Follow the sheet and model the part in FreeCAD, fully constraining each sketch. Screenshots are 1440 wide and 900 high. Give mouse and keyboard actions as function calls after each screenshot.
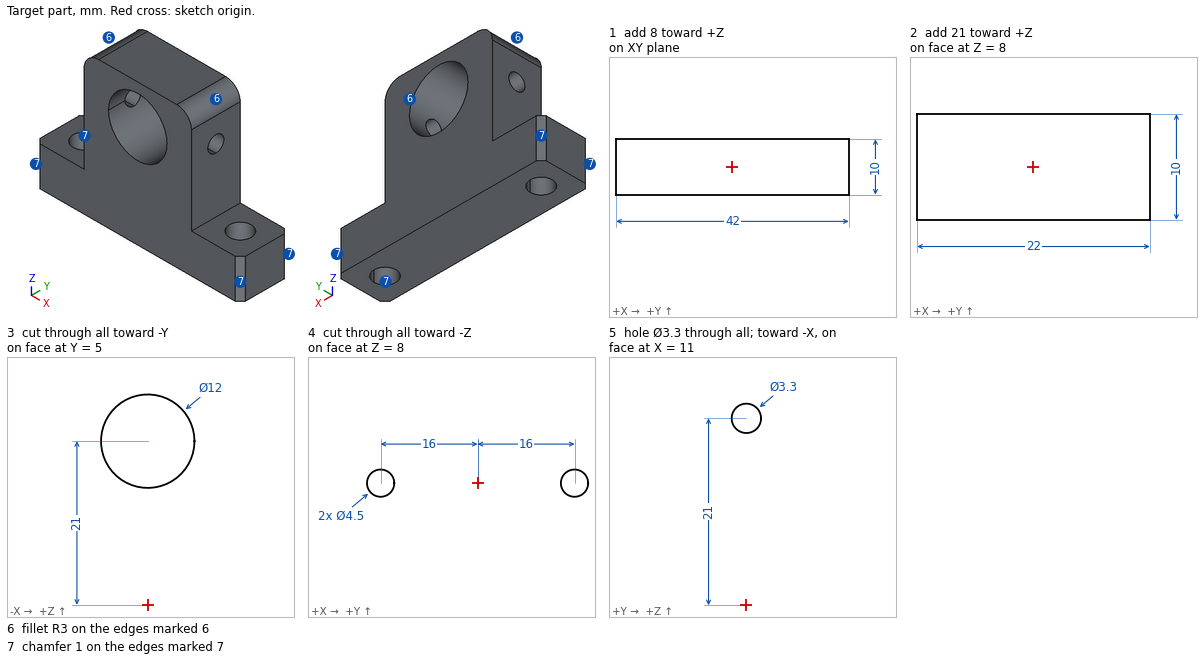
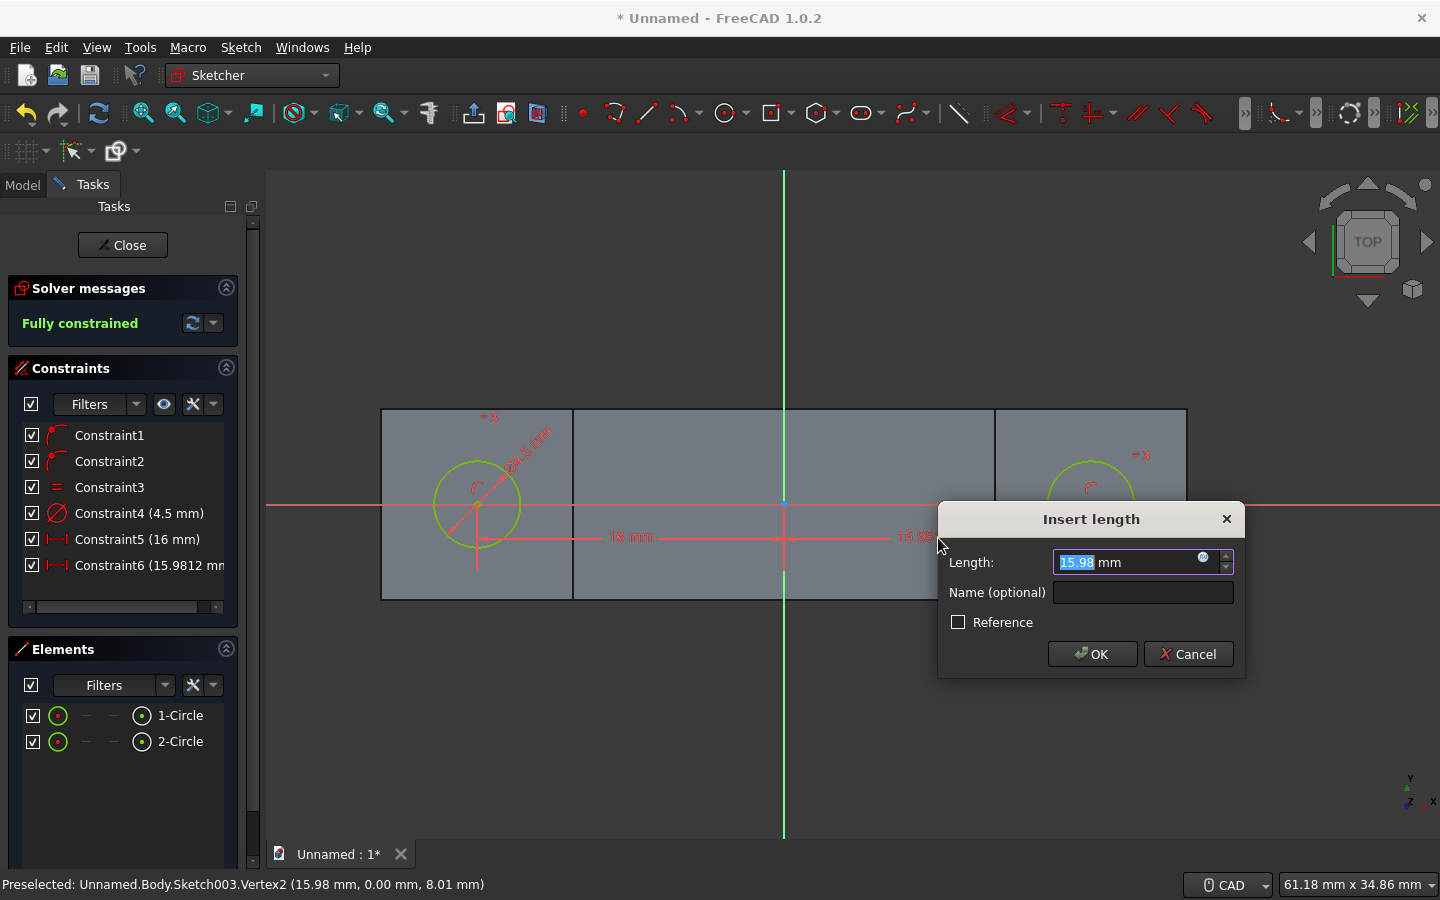
text(16)
key(Return)
key(Escape)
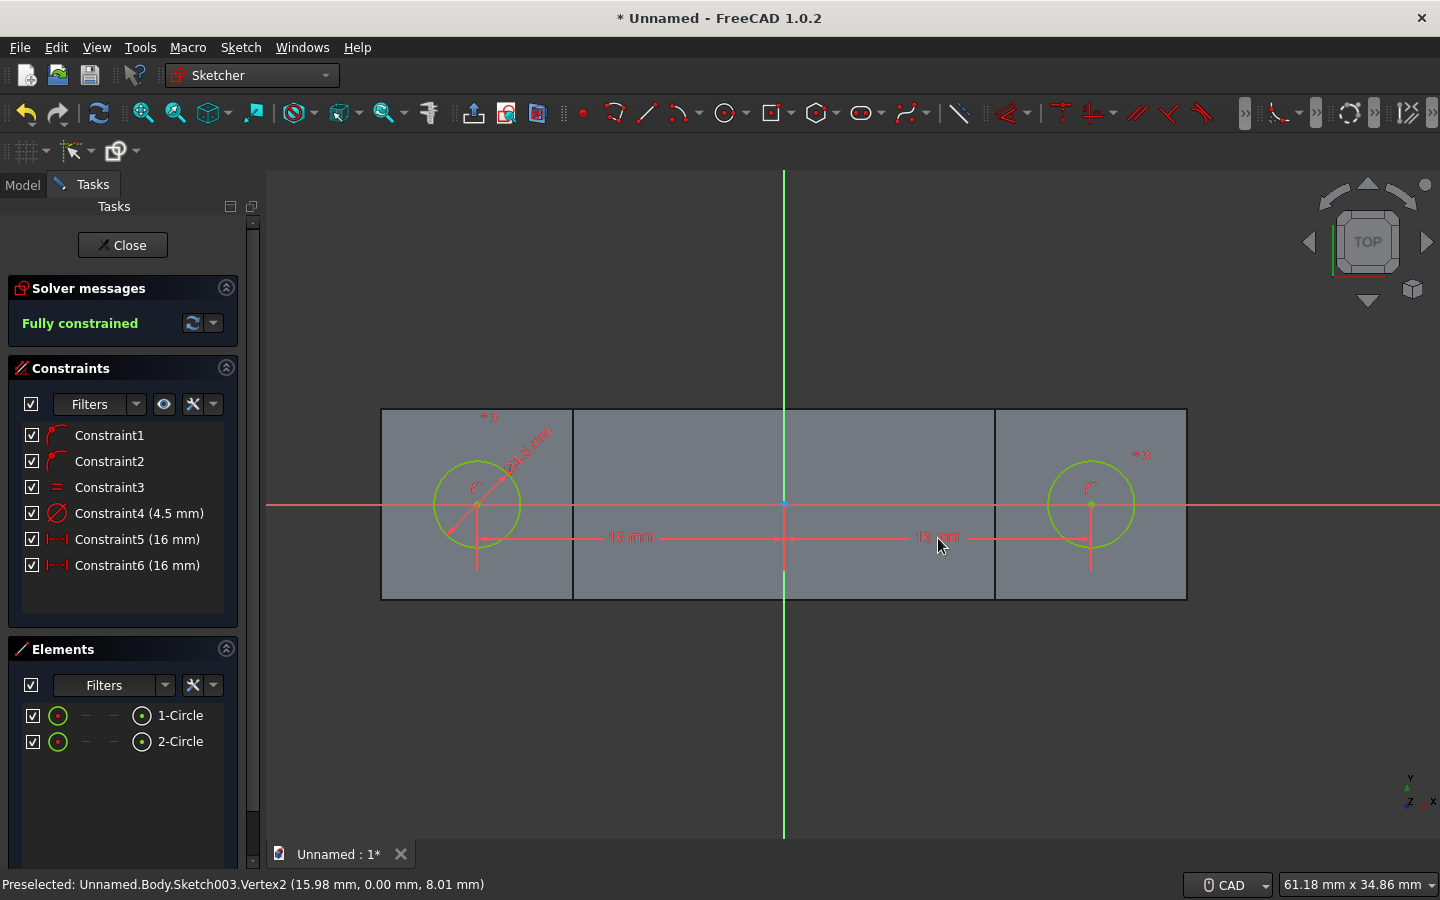
click(123, 245)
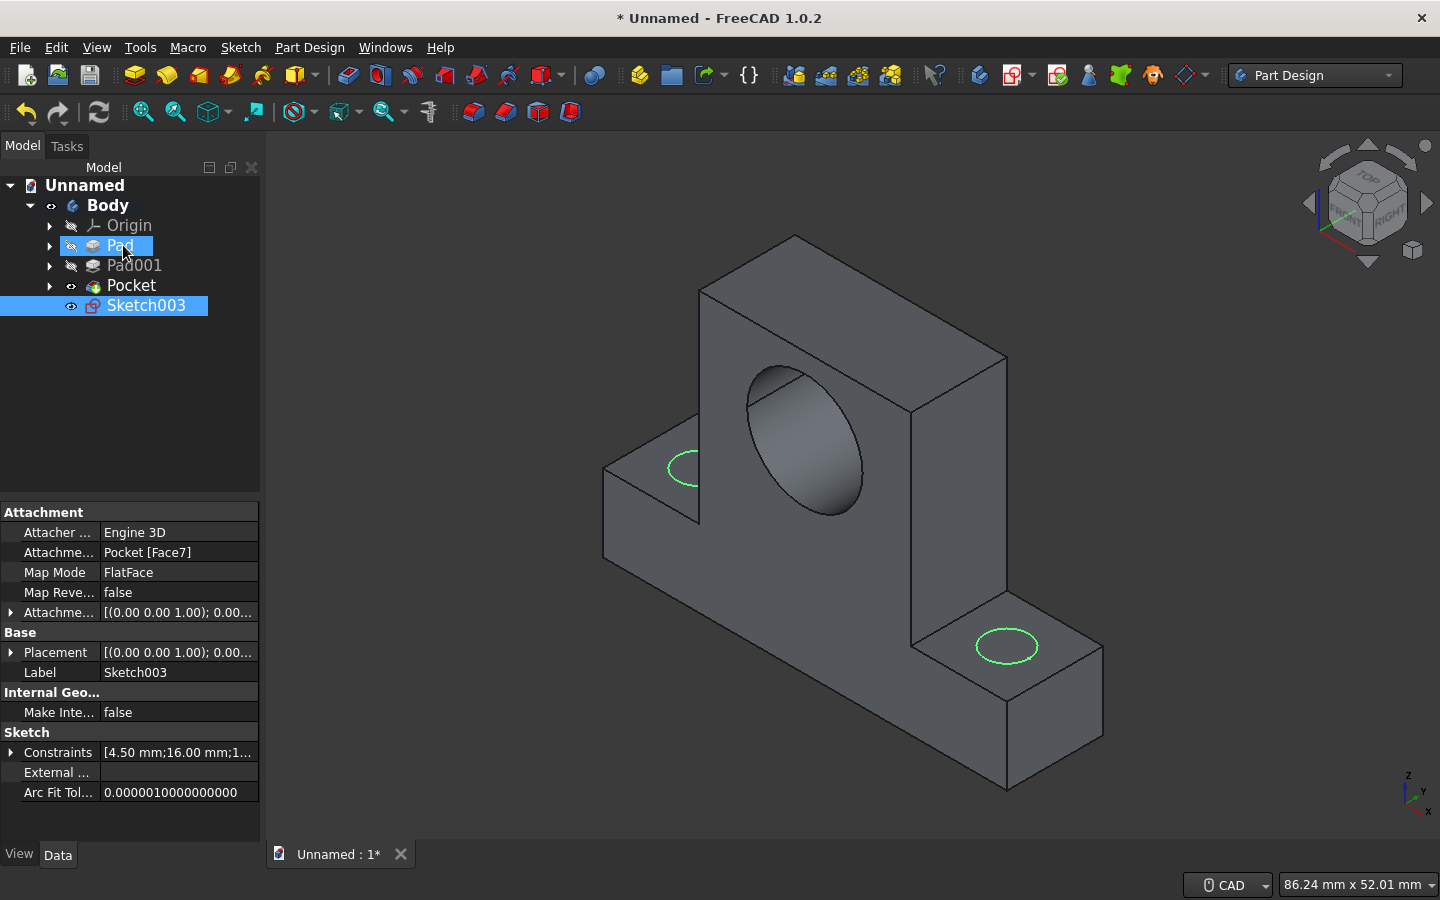
click(350, 76)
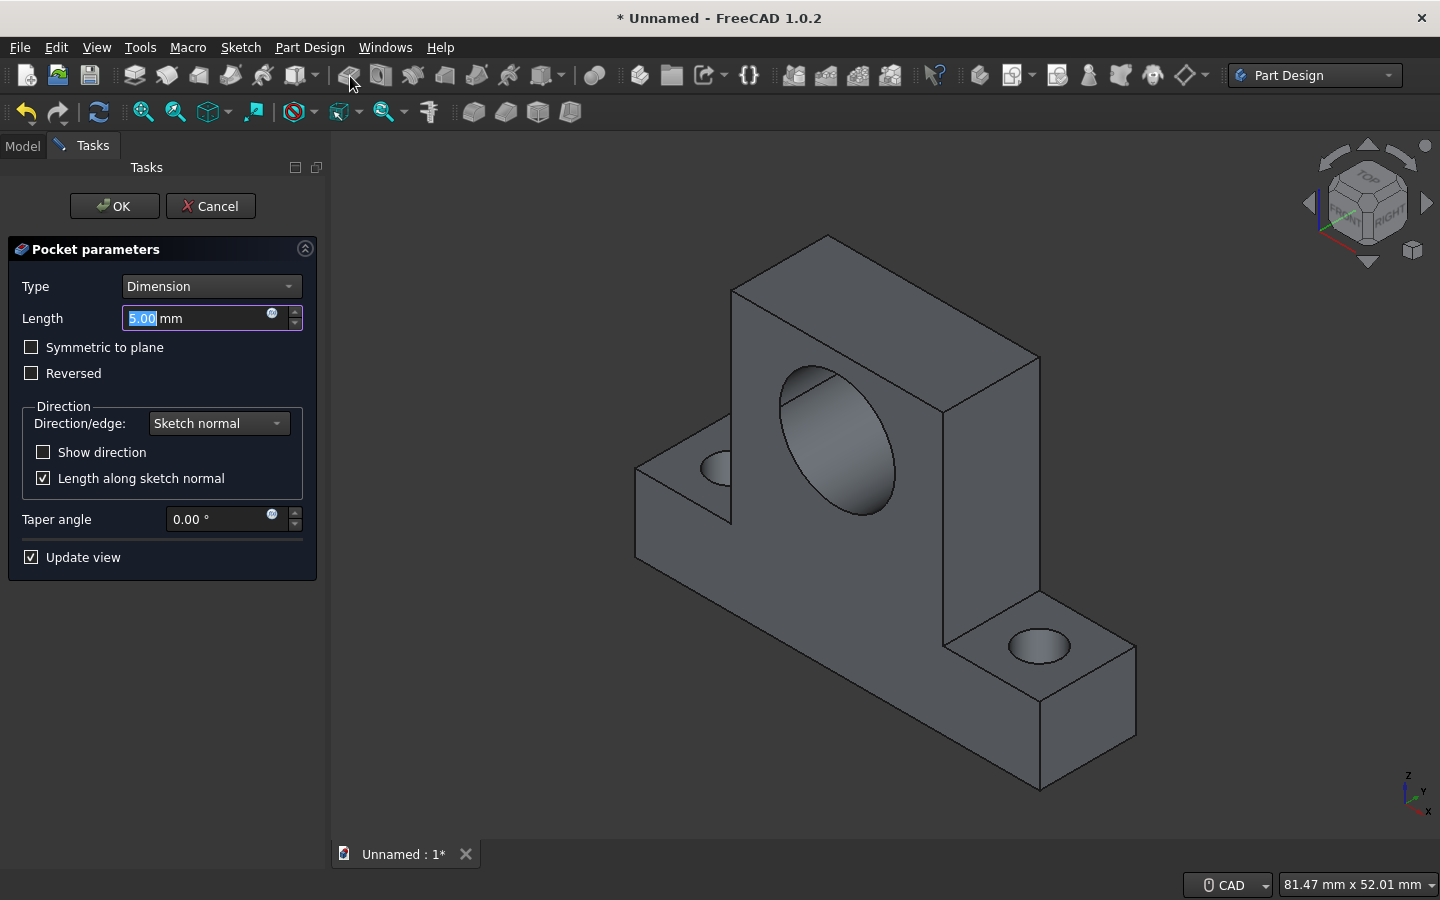
click(212, 286)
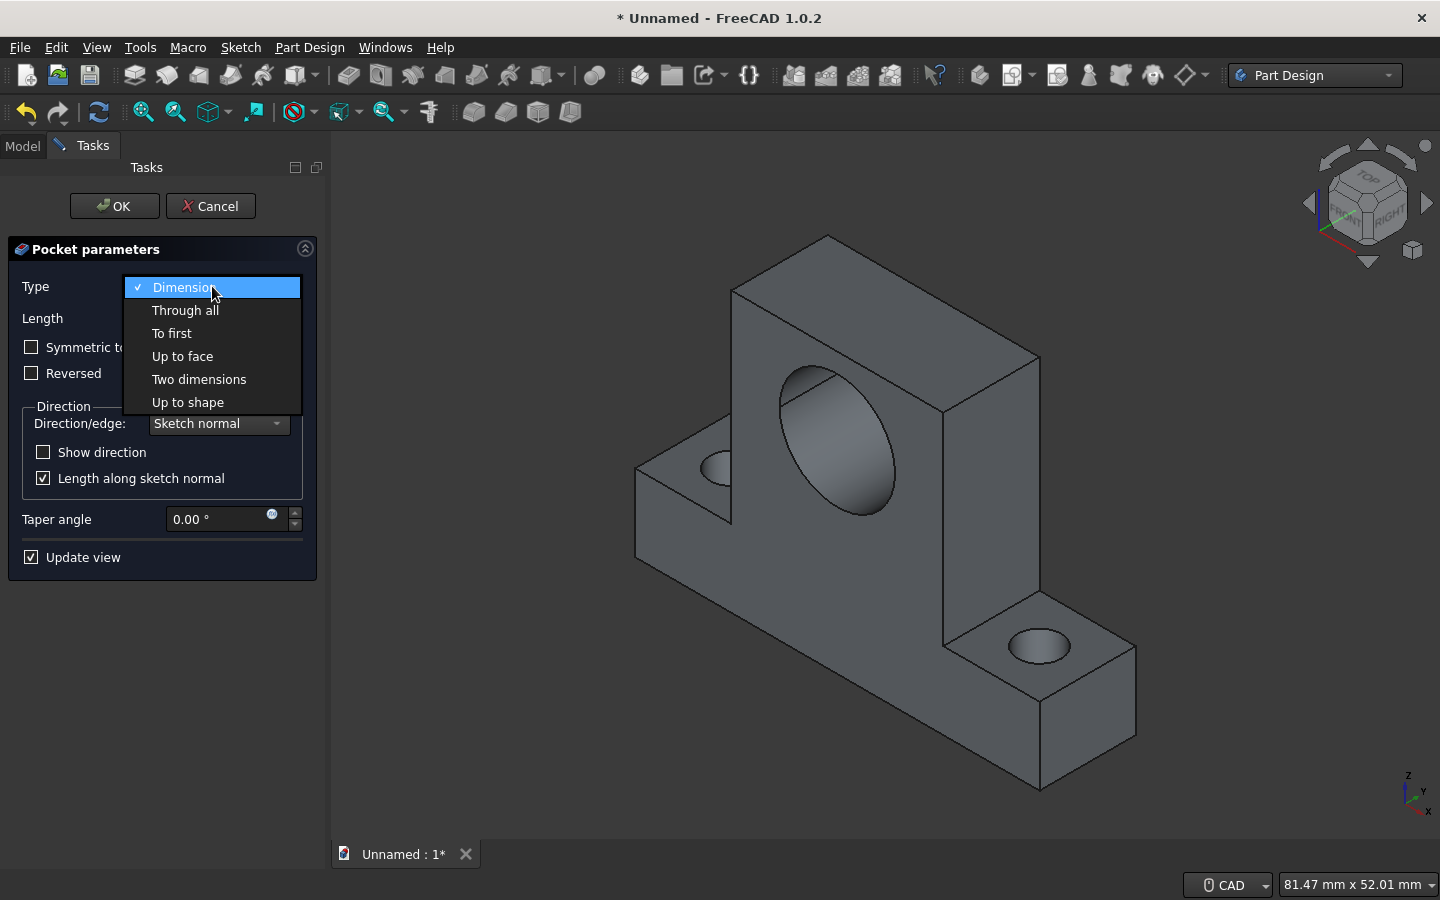
click(212, 310)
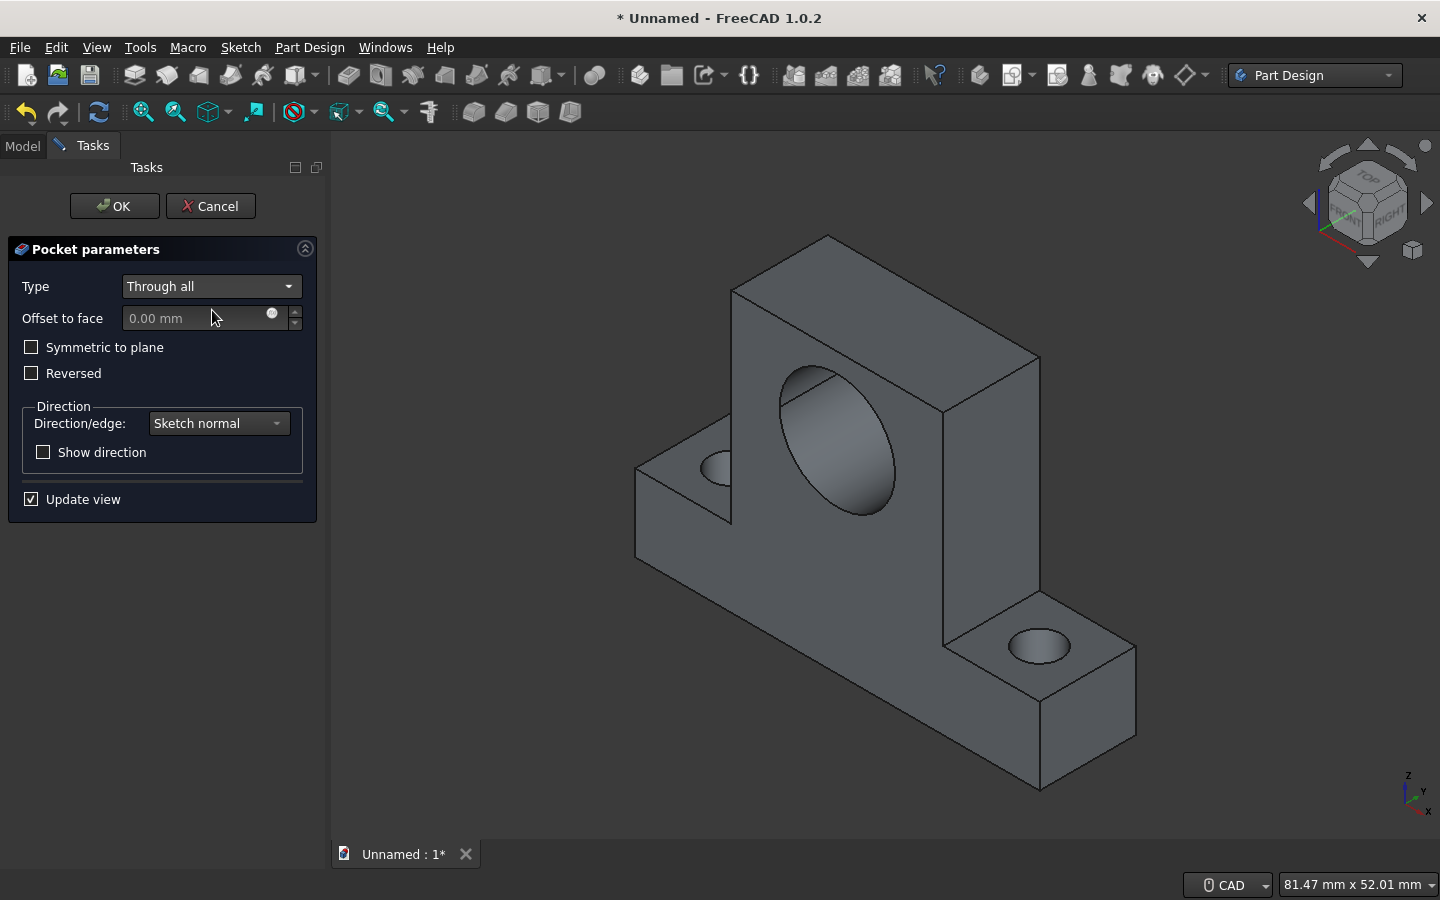
click(115, 206)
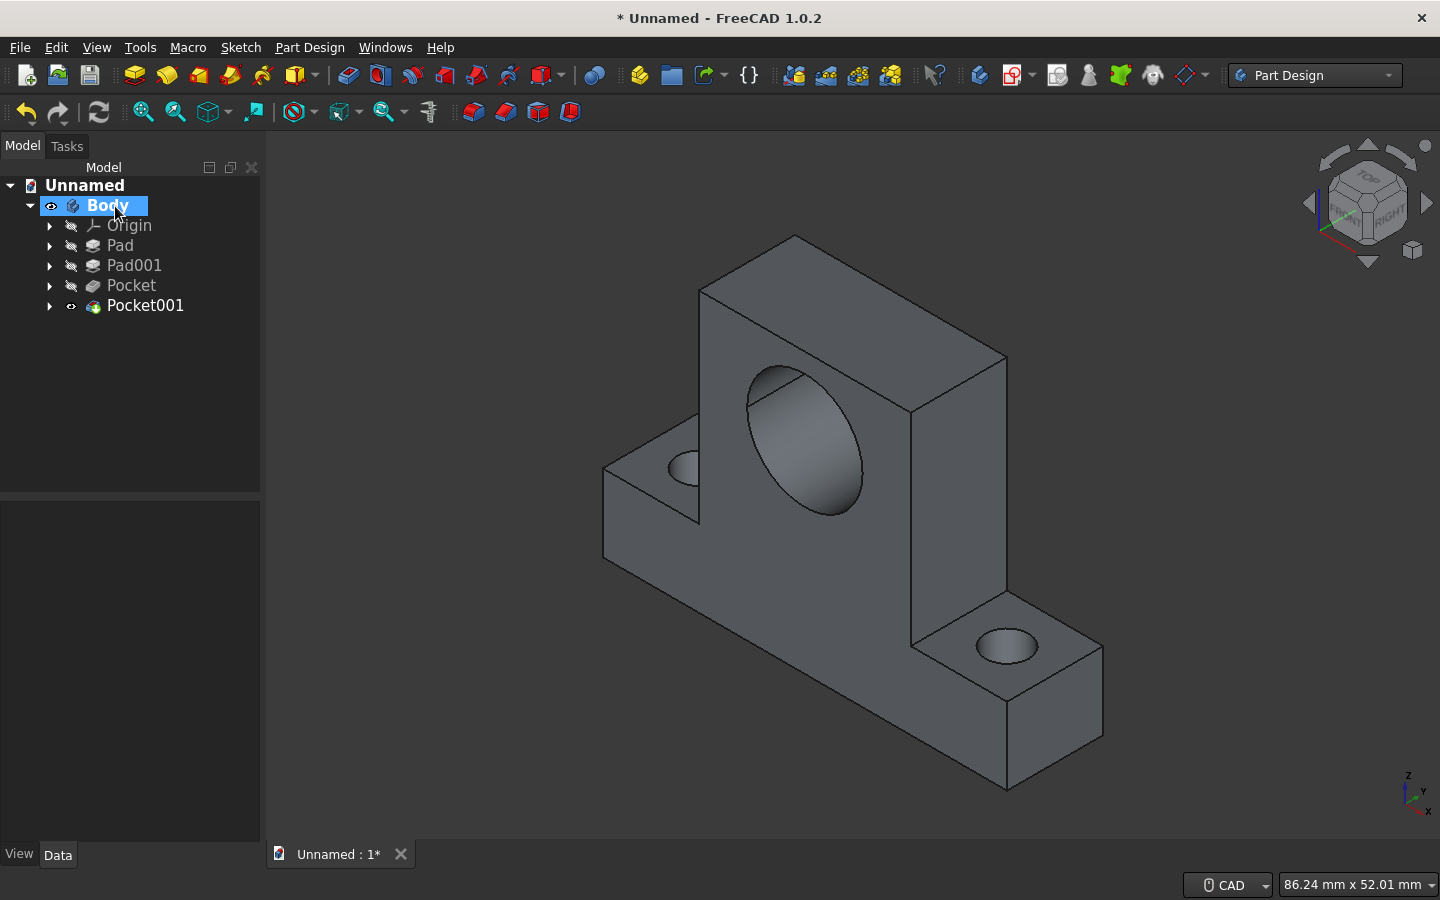
click(959, 467)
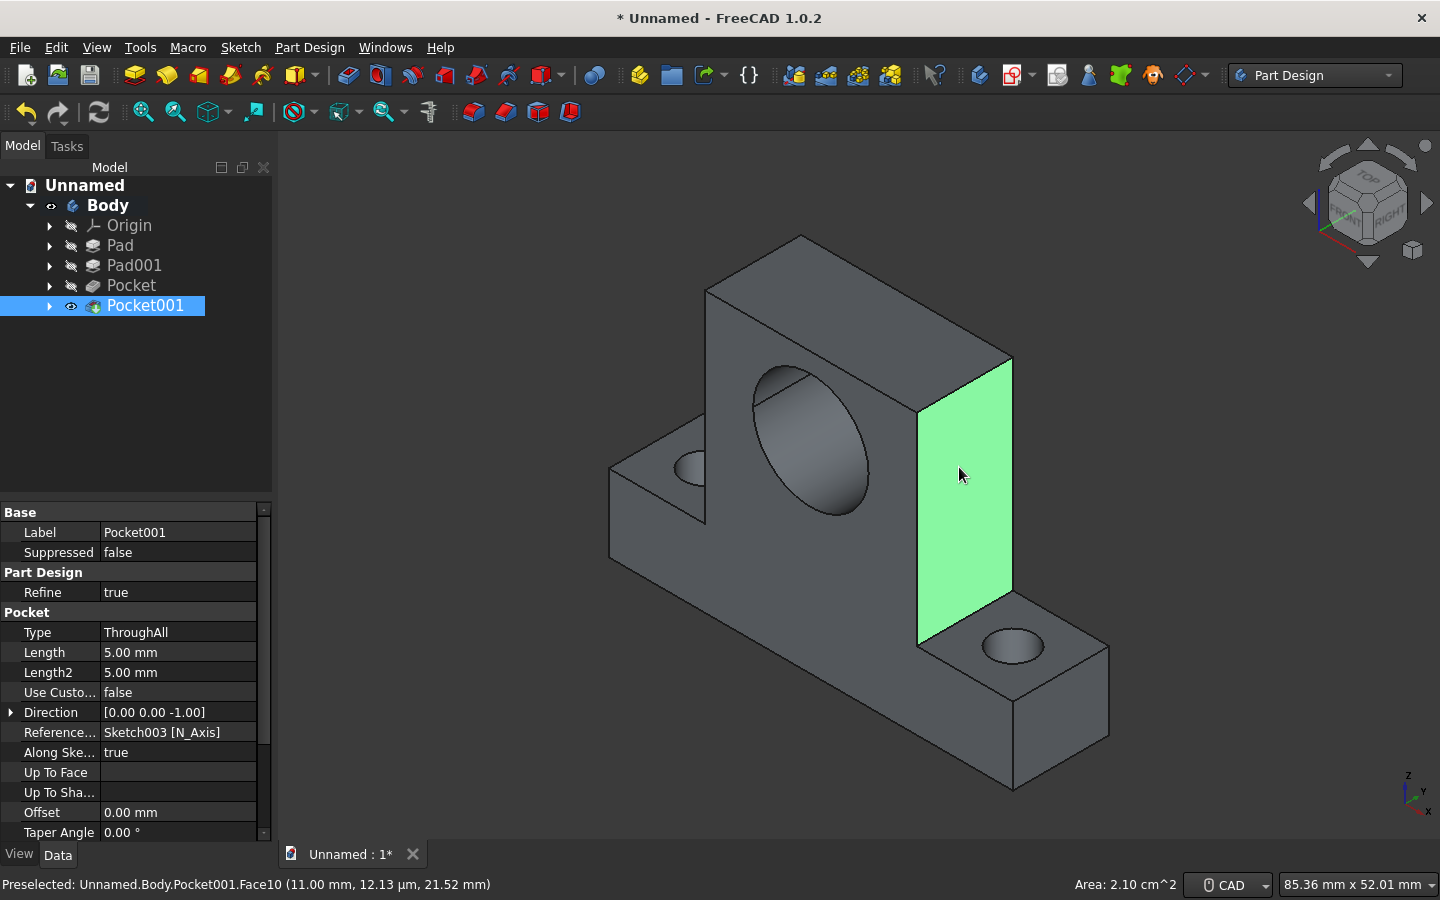
click(1012, 76)